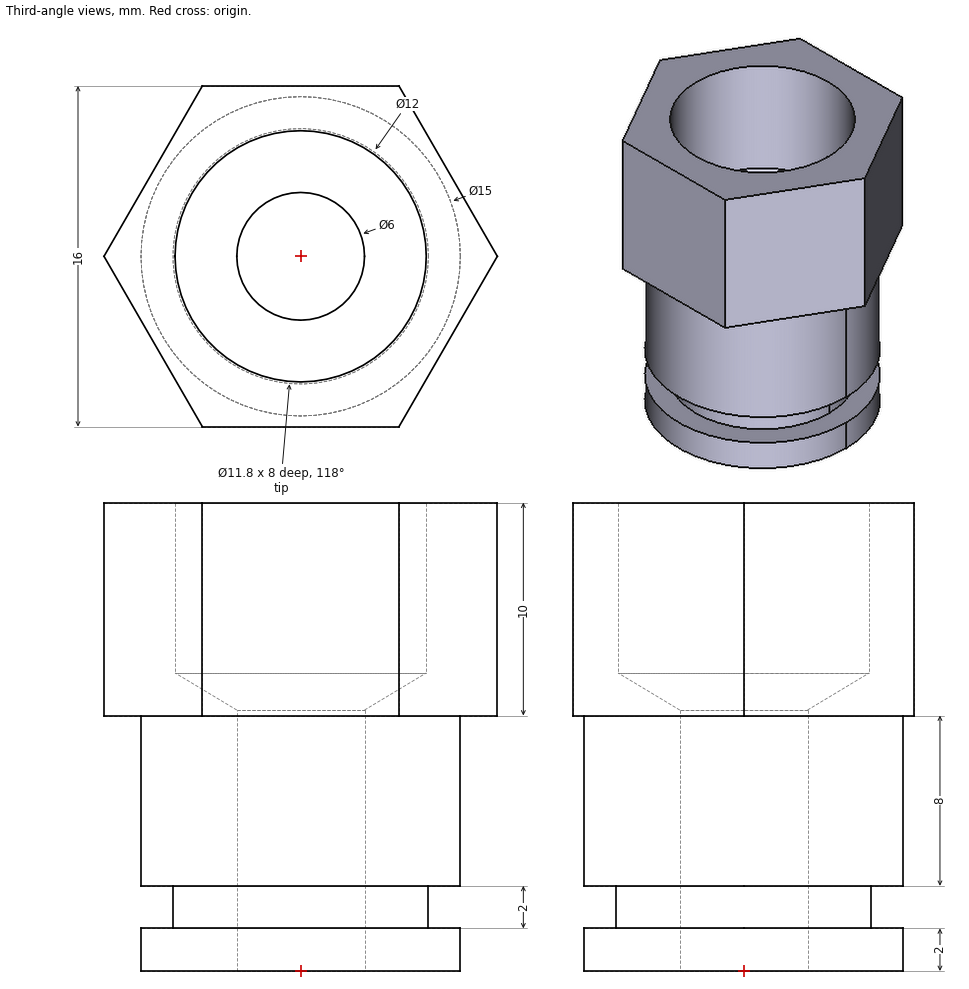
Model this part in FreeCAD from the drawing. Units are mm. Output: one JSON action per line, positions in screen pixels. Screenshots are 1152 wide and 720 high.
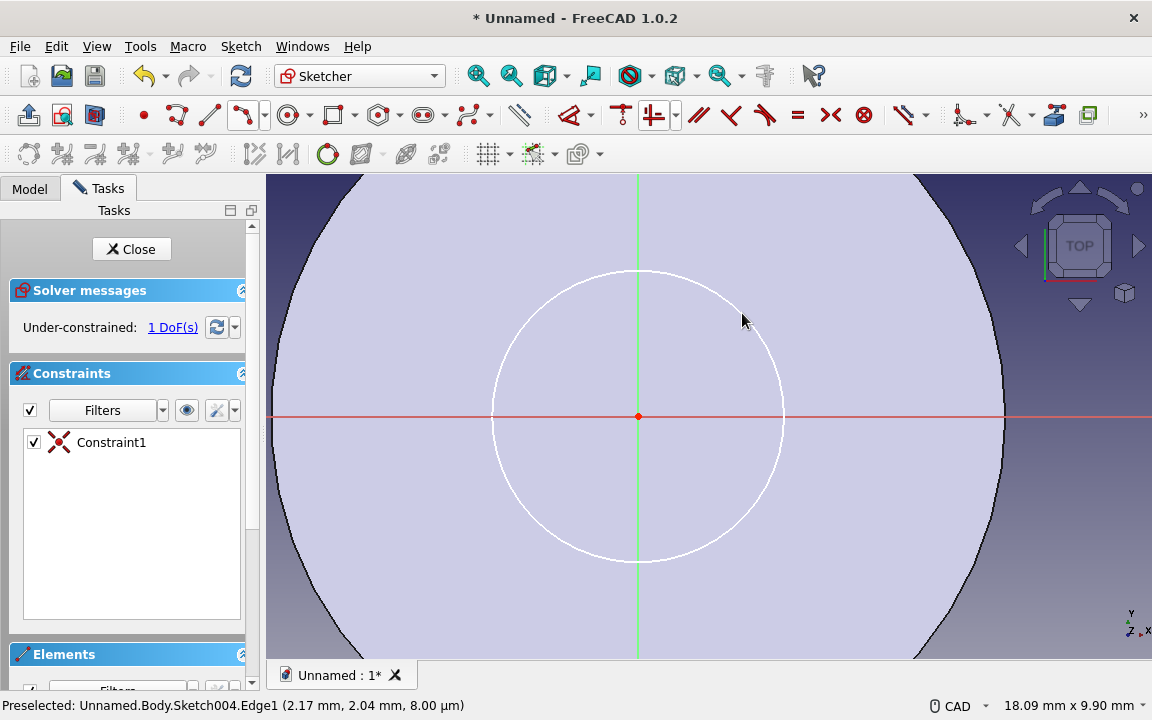
{"action": "key", "text": "d"}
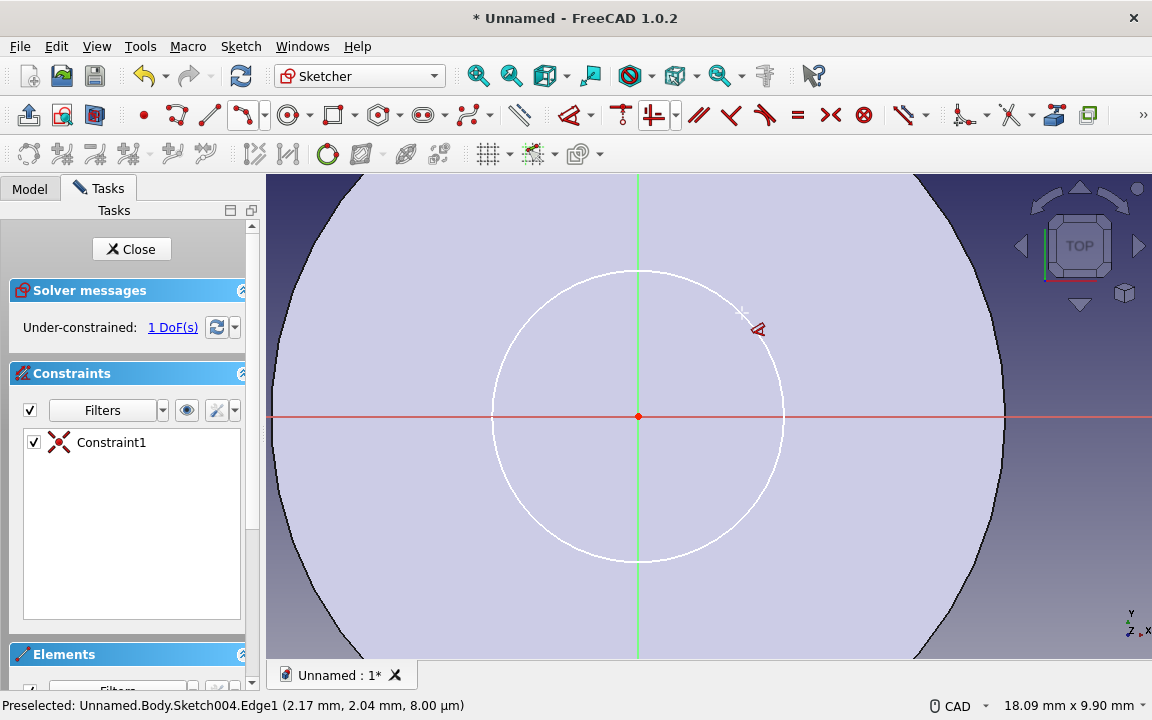
{"action": "left_click", "coordinate": [741, 313]}
{"action": "left_click", "coordinate": [764, 290]}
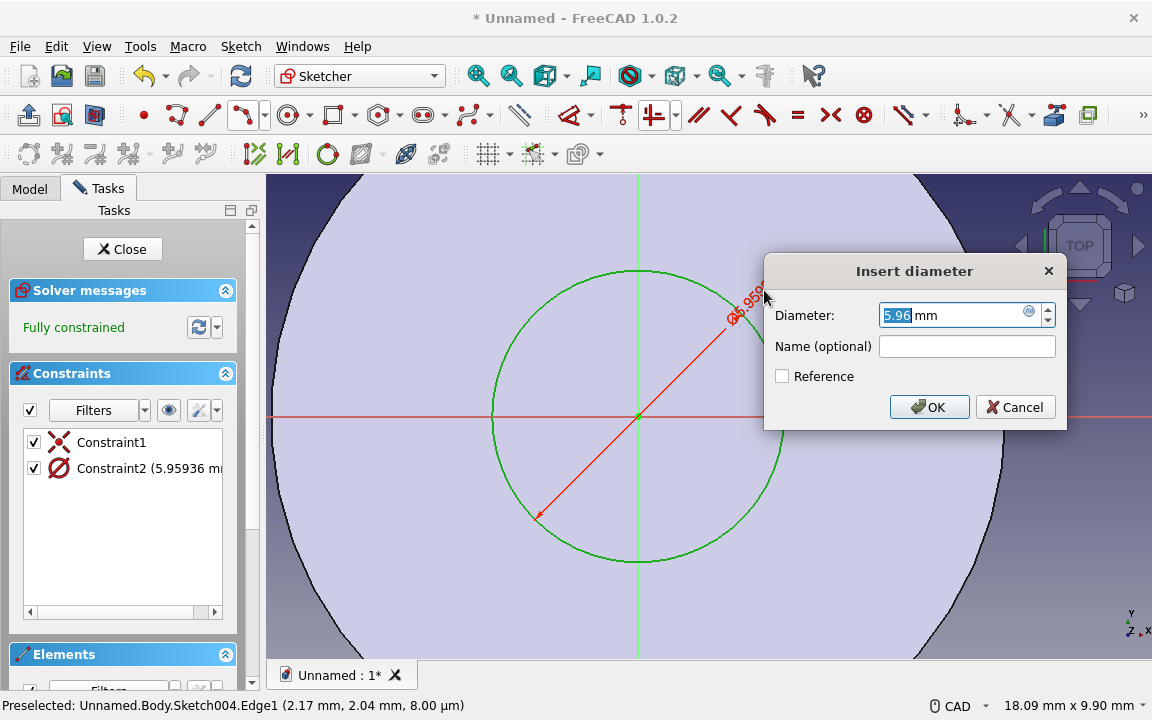
{"action": "type", "text": "6"}
{"action": "key", "text": "Return"}
{"action": "key", "text": "Escape"}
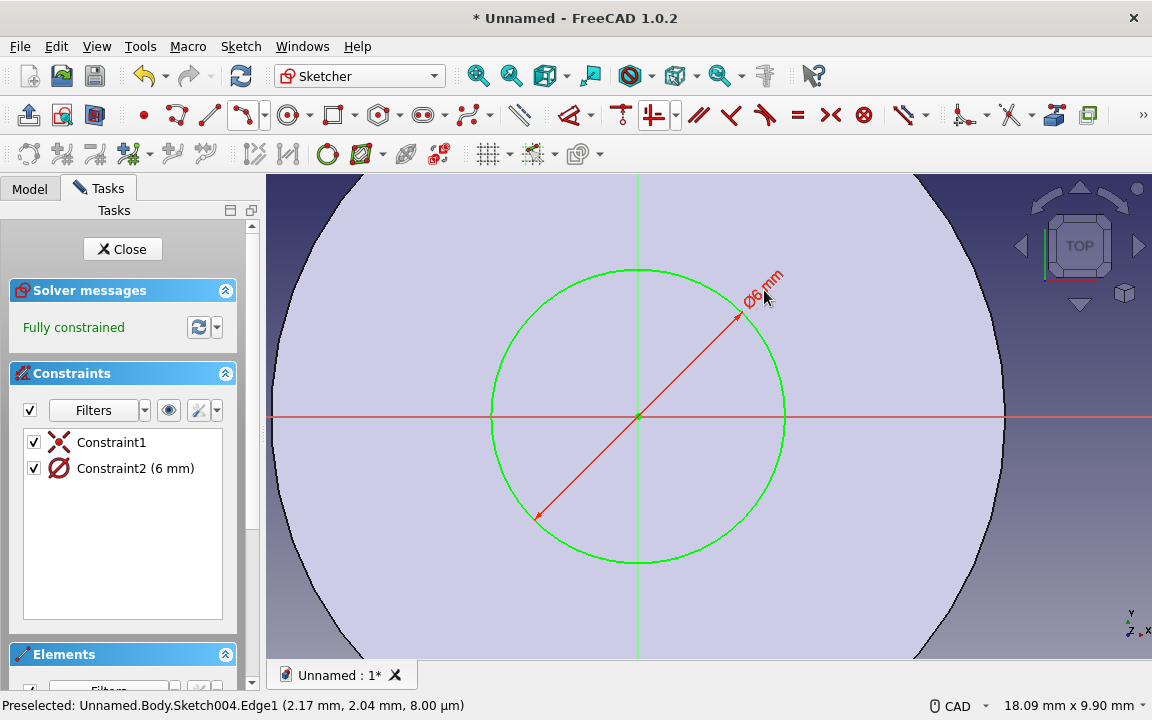
{"action": "left_click", "coordinate": [123, 249]}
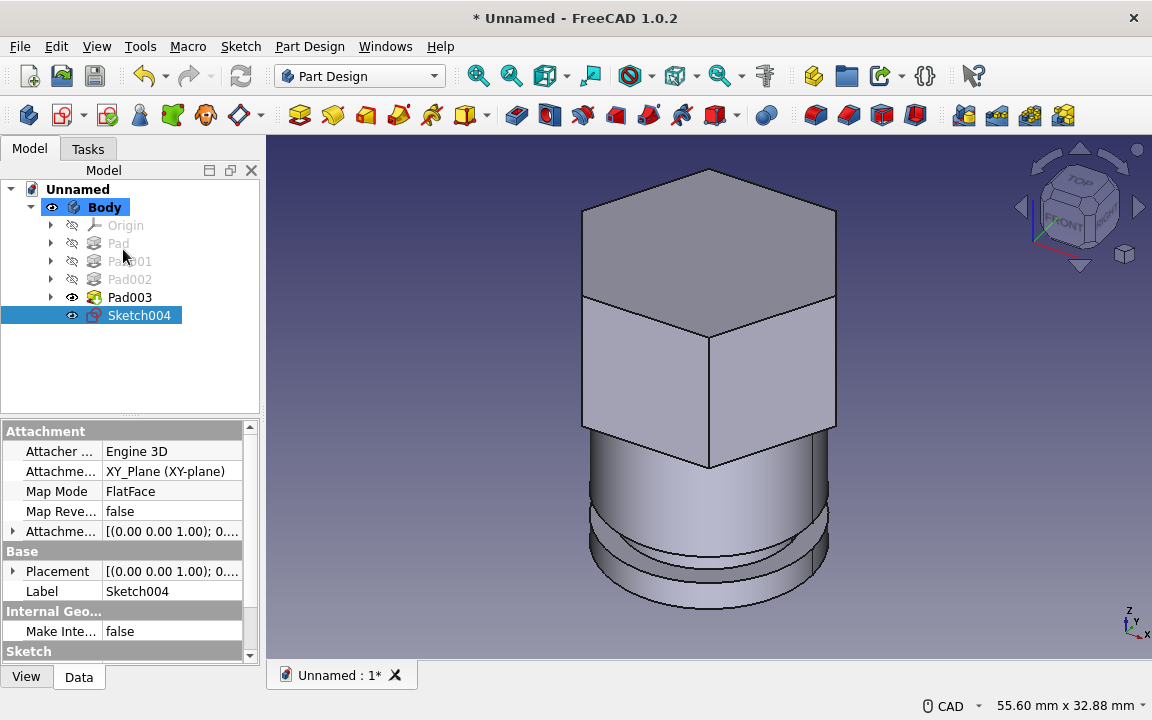
{"action": "left_click", "coordinate": [517, 116]}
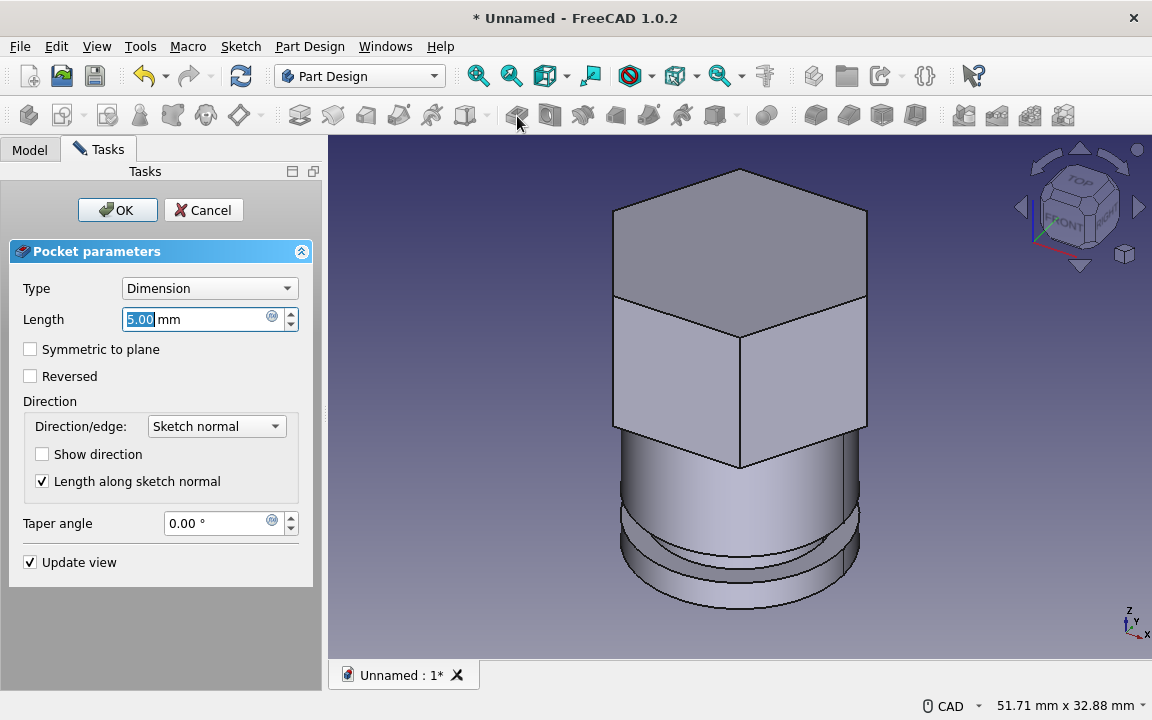
{"action": "left_click", "coordinate": [210, 288]}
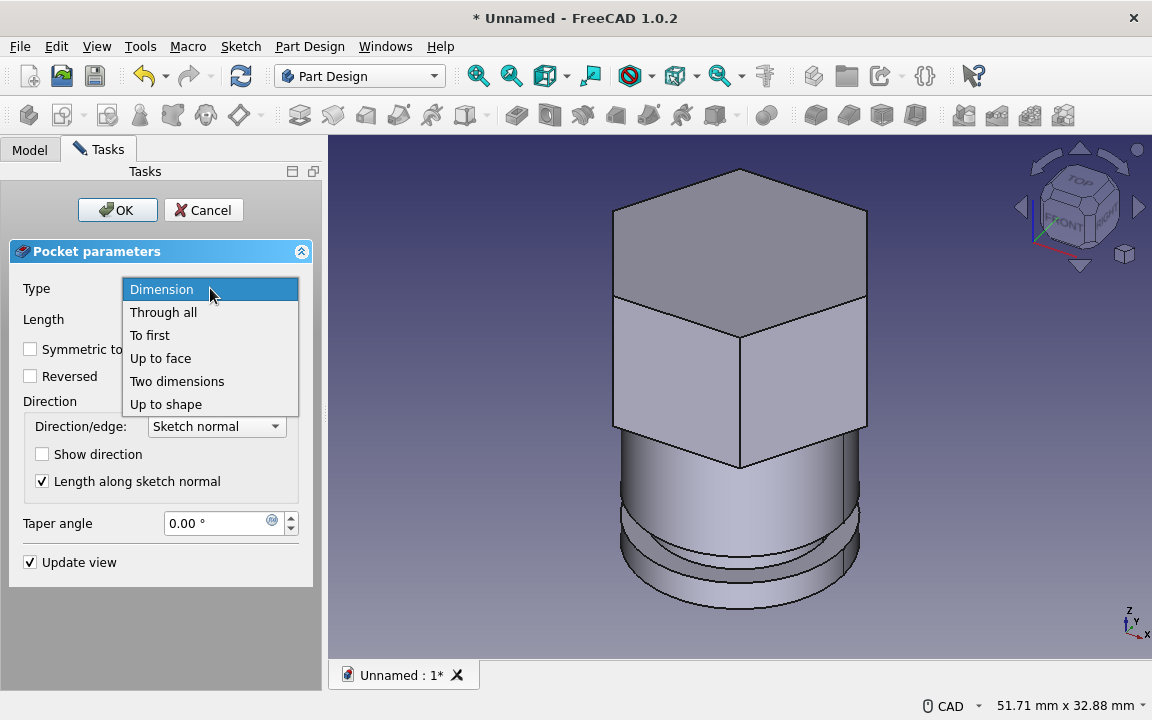
{"action": "left_click", "coordinate": [208, 312]}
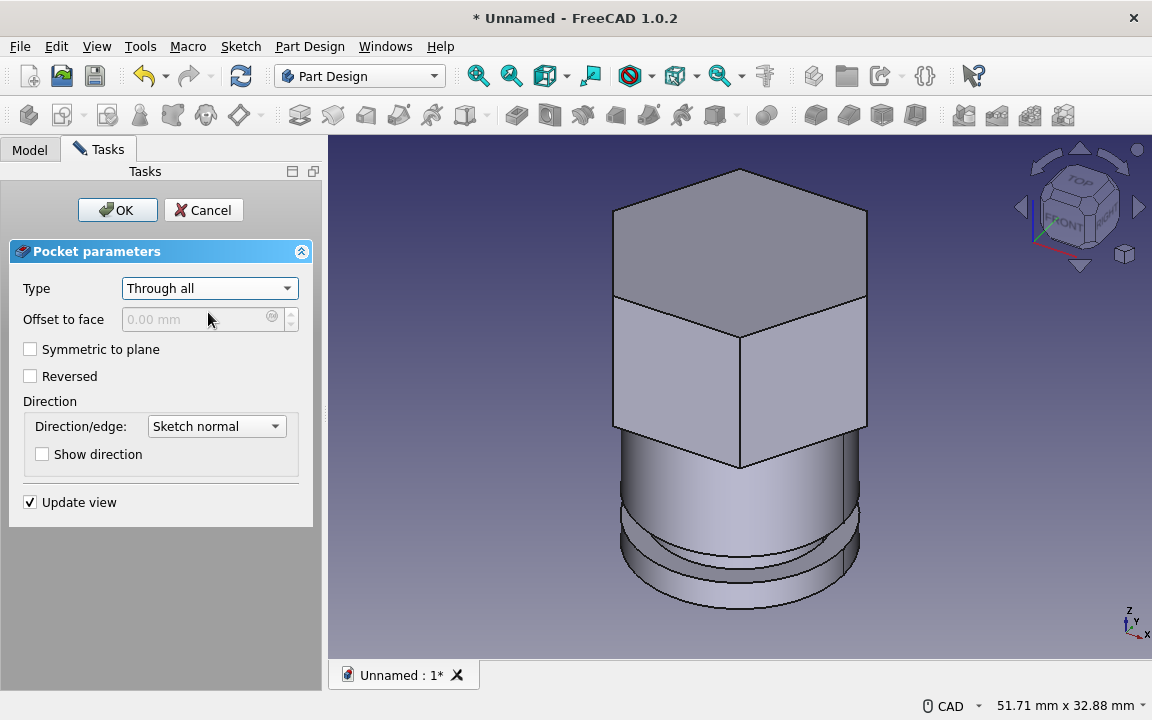
{"action": "left_click", "coordinate": [31, 376]}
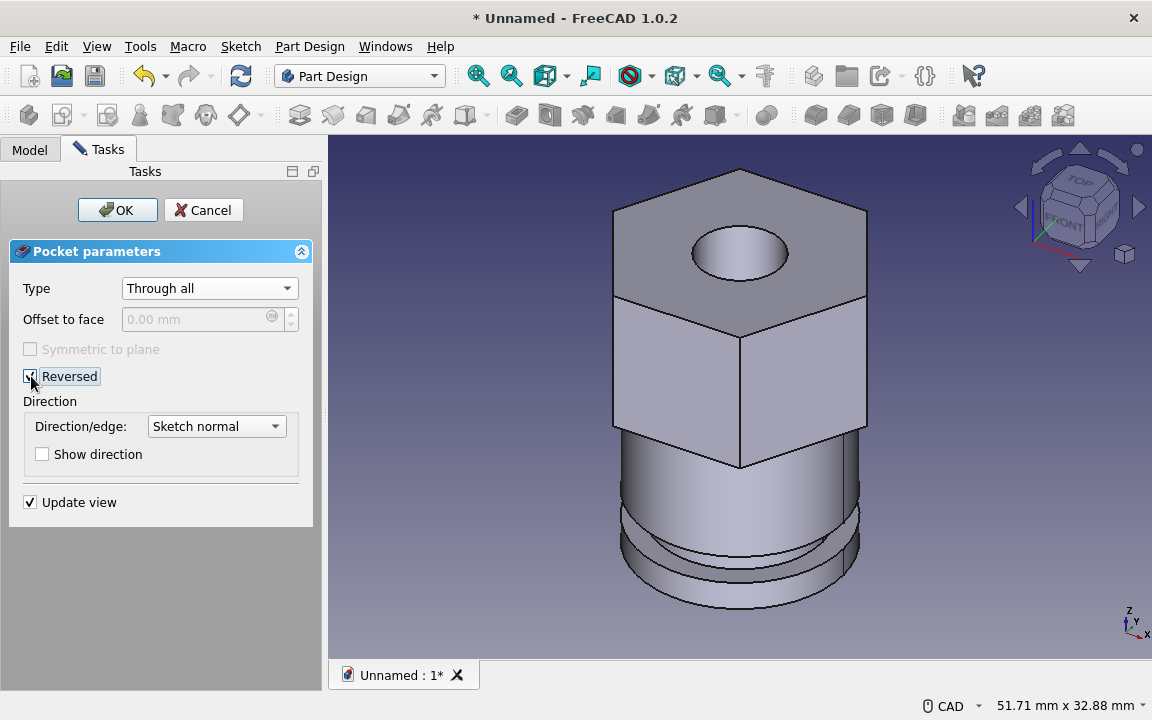
{"action": "left_click", "coordinate": [118, 210]}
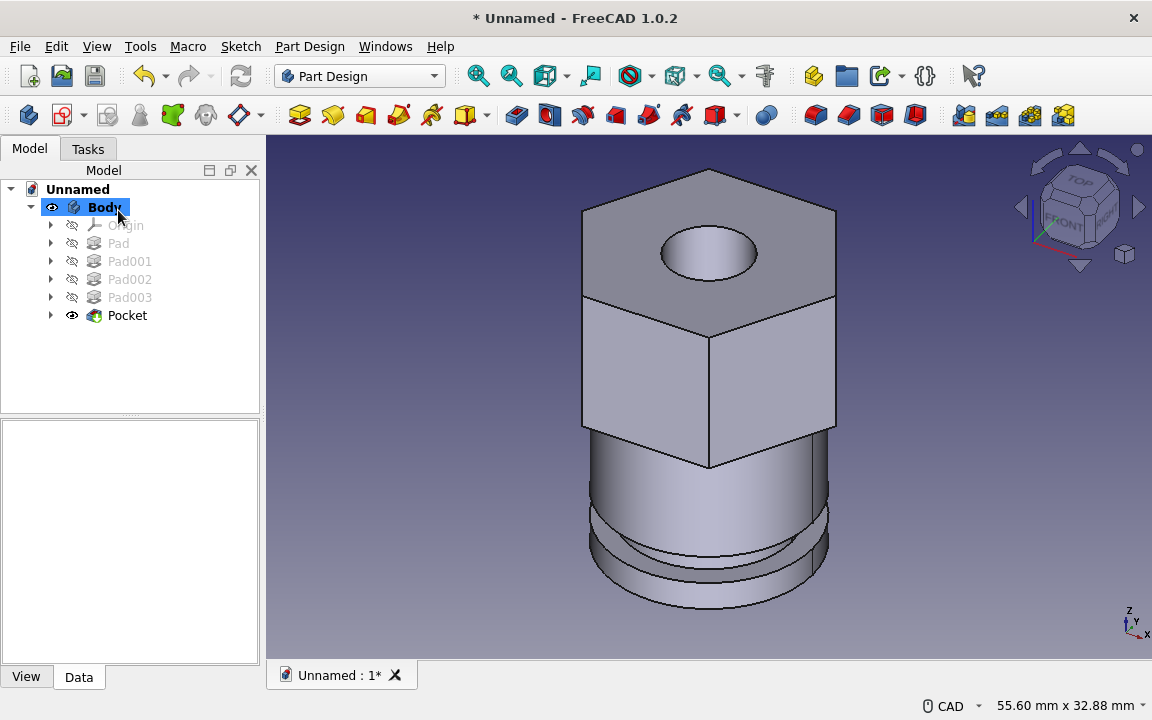
{"action": "left_click", "coordinate": [654, 210]}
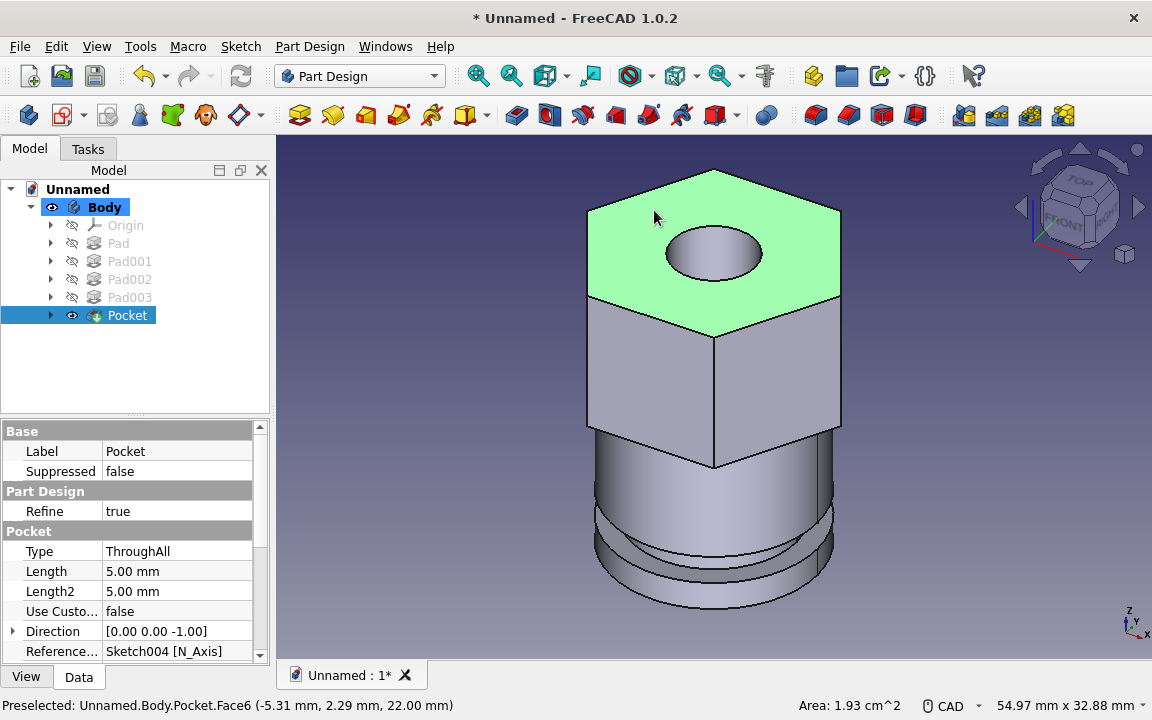
{"action": "left_click", "coordinate": [62, 116]}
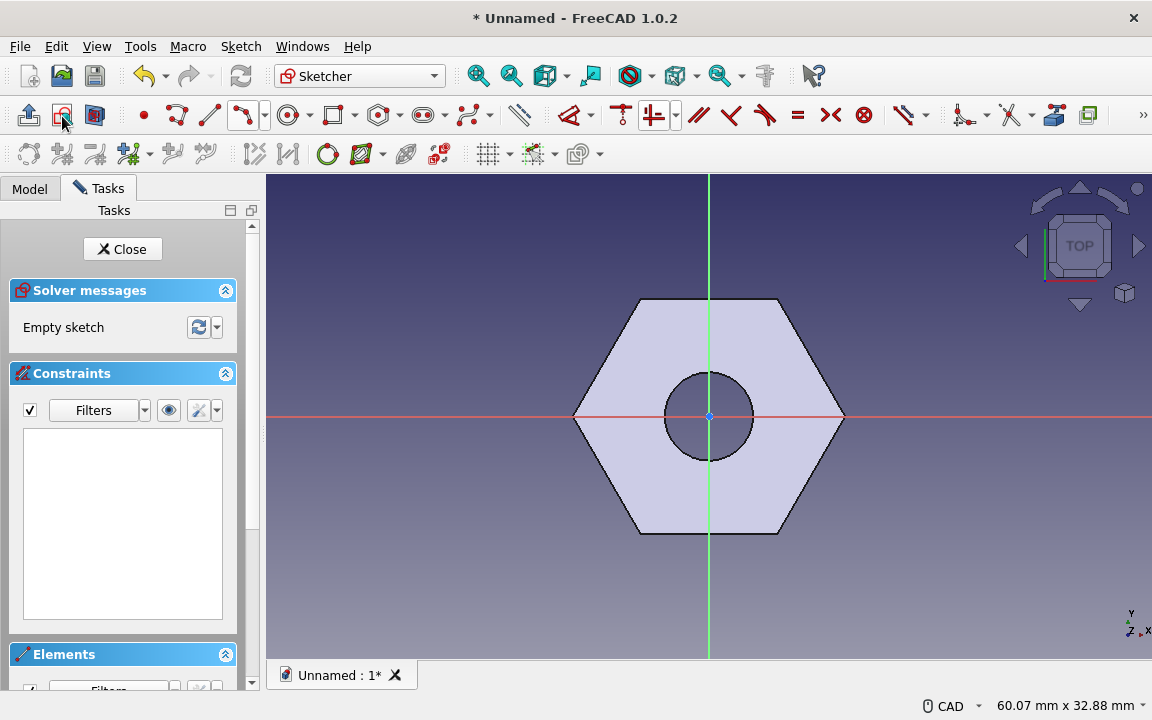
{"action": "scroll", "coordinate": [792, 416], "scroll_direction": "up", "scroll_amount": 3}